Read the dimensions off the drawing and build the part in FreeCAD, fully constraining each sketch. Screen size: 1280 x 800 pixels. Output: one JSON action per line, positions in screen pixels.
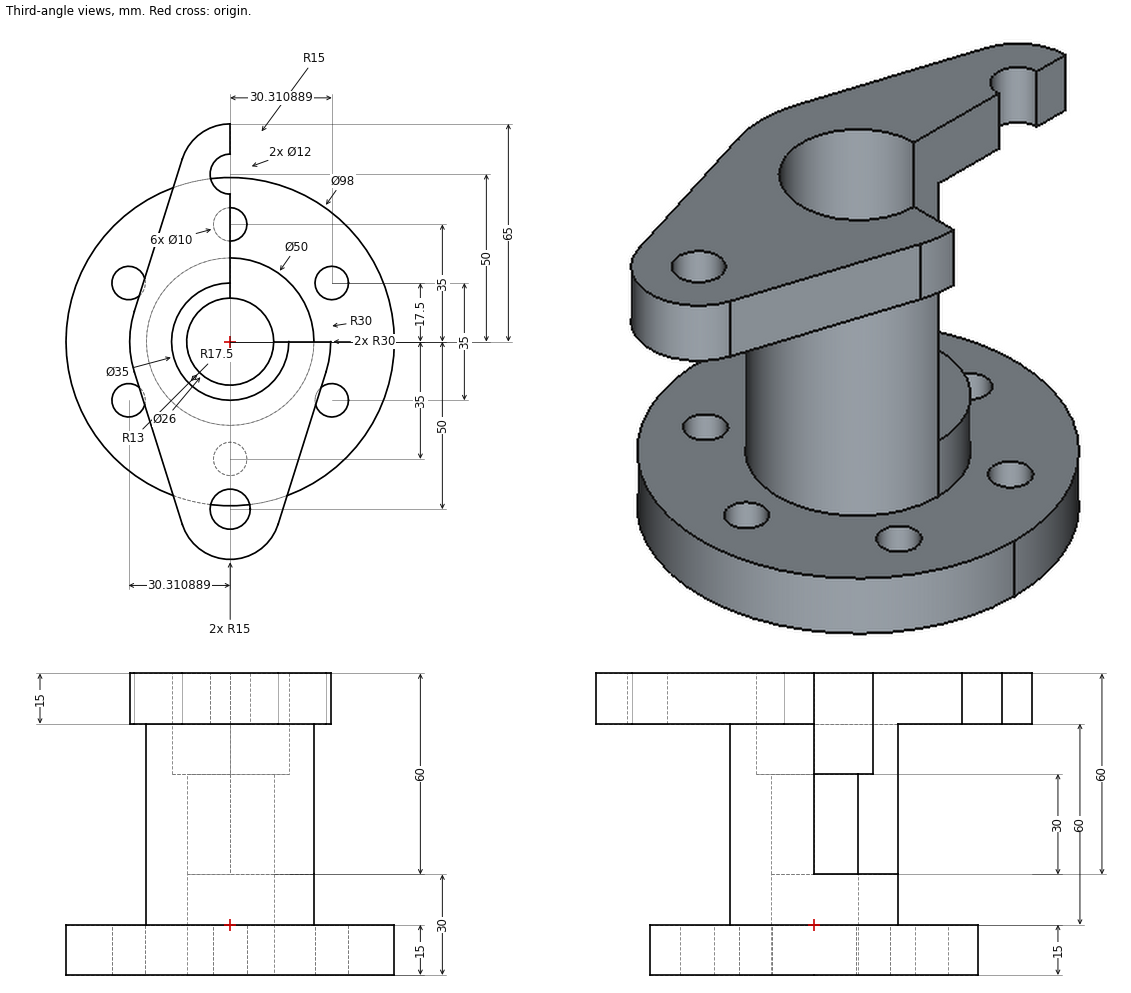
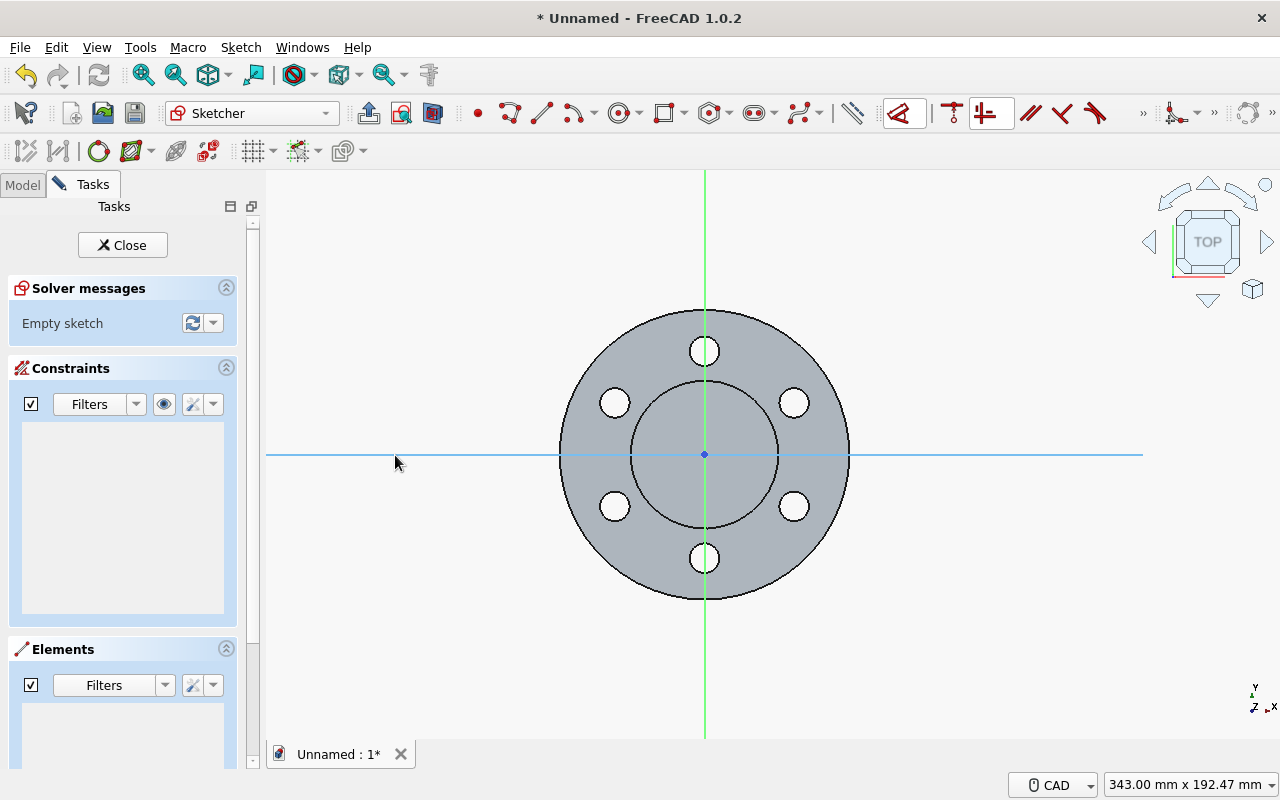
{"action": "left_click", "coordinate": [542, 114]}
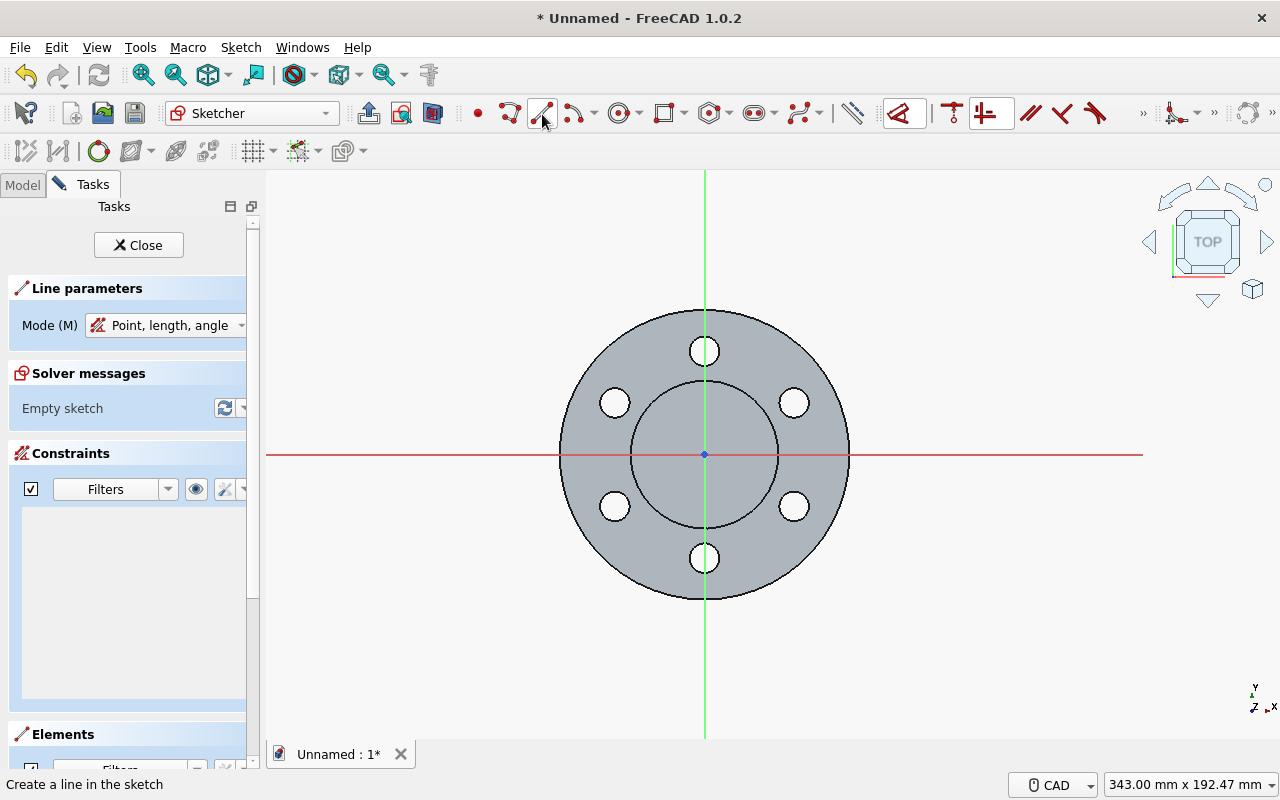
{"action": "left_click", "coordinate": [620, 481]}
{"action": "left_click", "coordinate": [662, 616]}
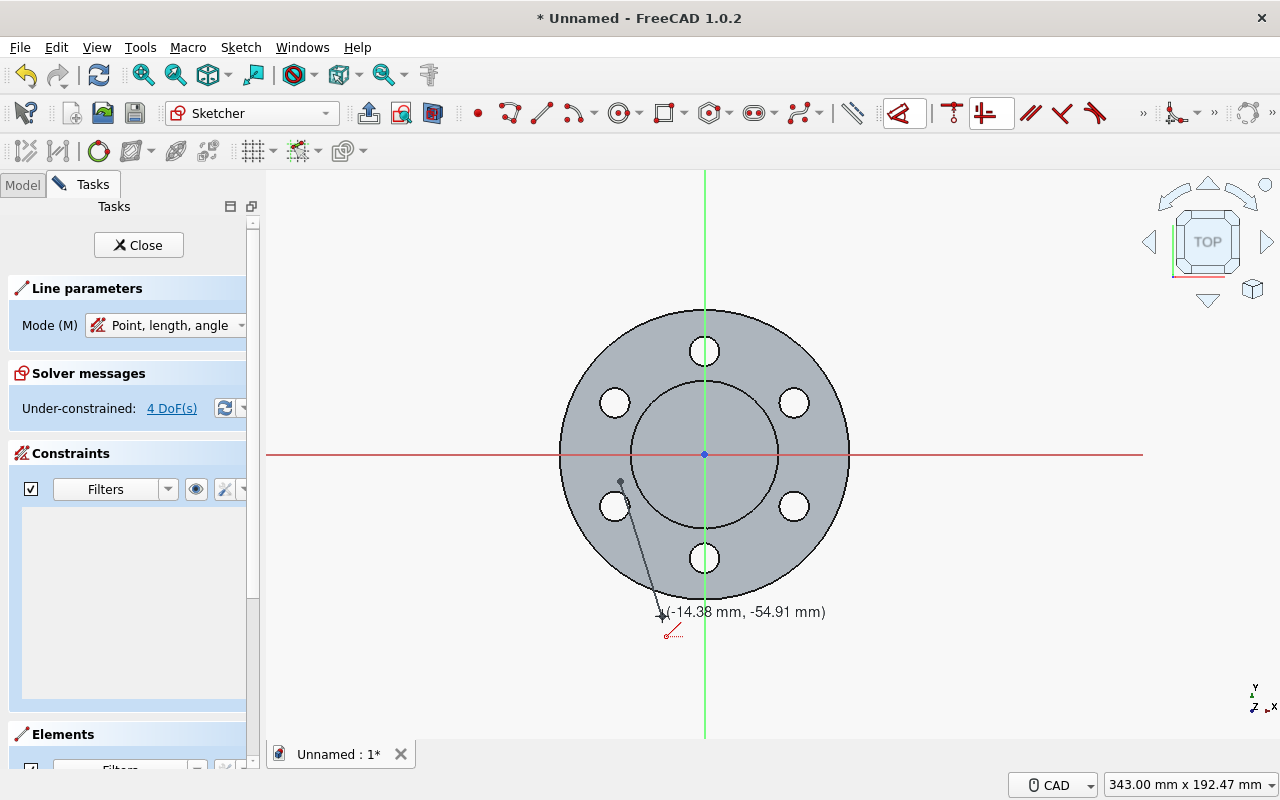
{"action": "left_click", "coordinate": [747, 616]}
{"action": "left_click", "coordinate": [789, 481]}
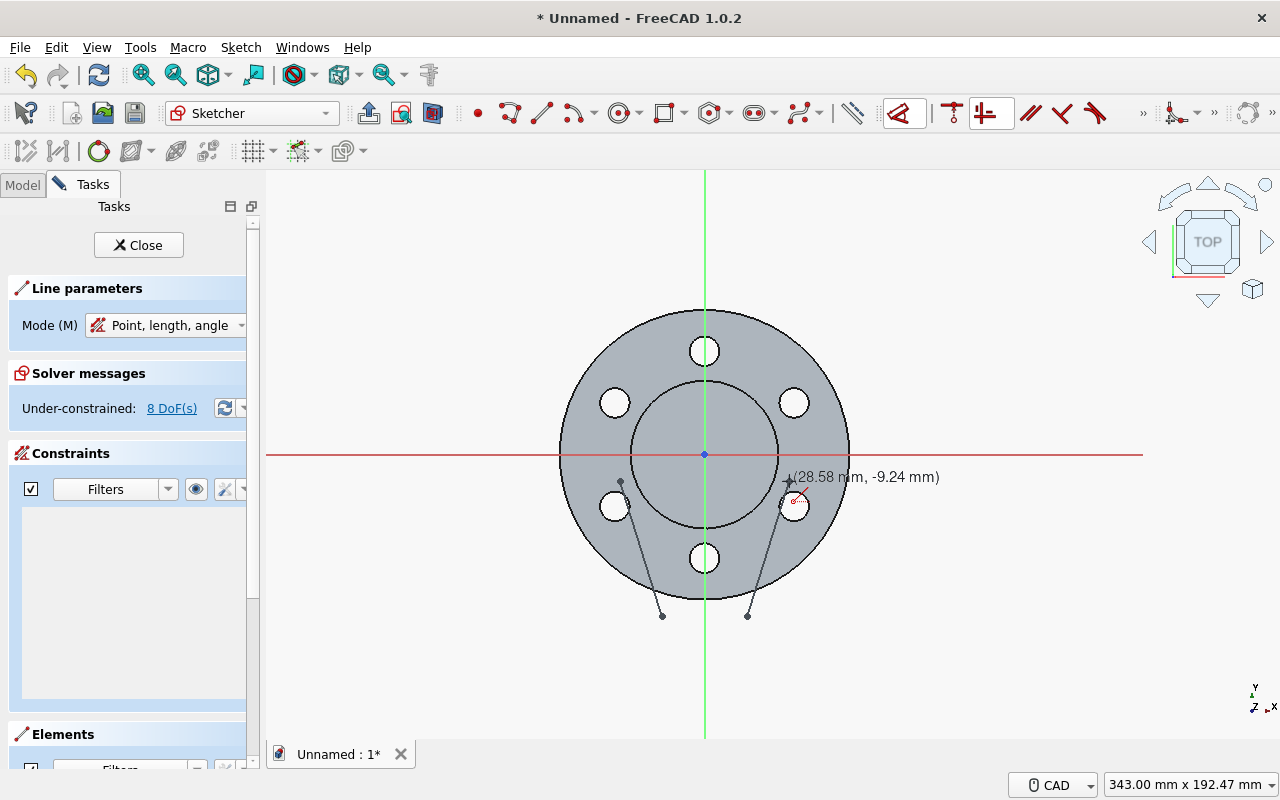
{"action": "left_click", "coordinate": [789, 428]}
{"action": "left_click", "coordinate": [747, 294]}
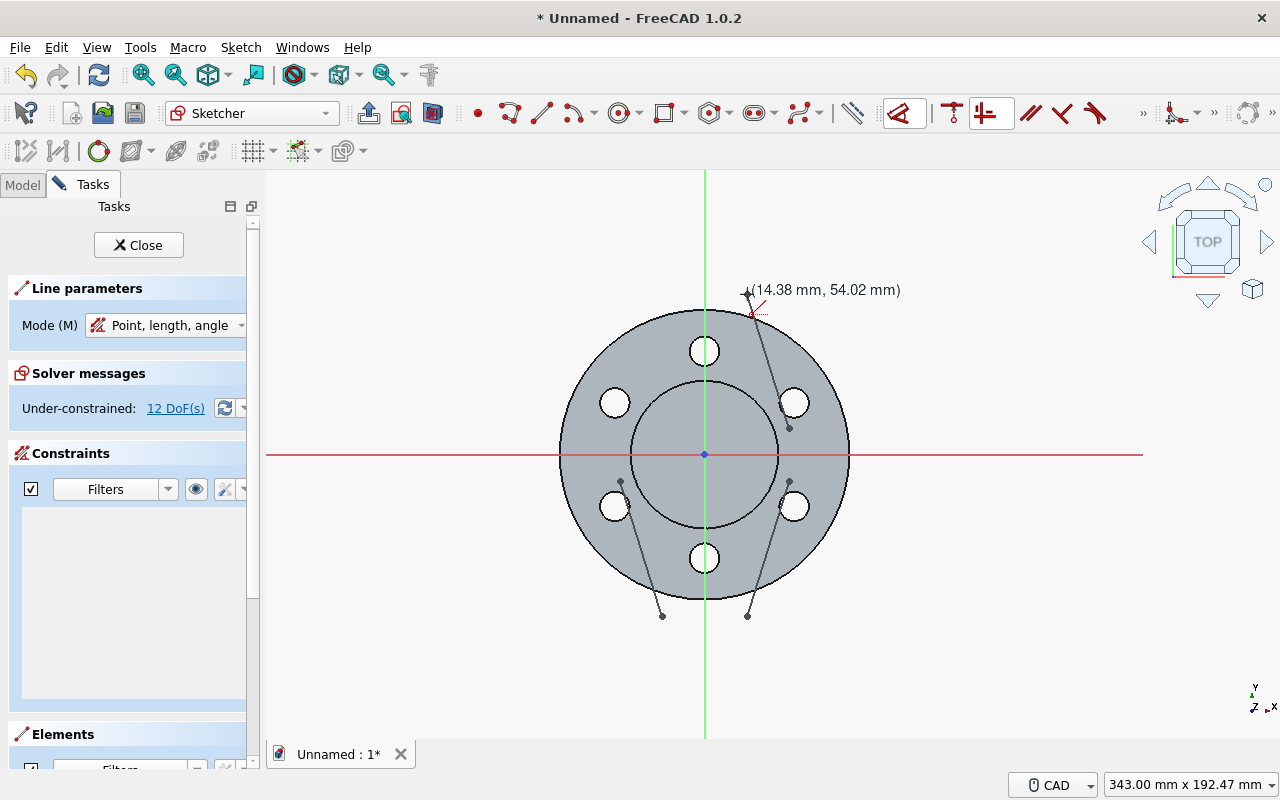
{"action": "left_click", "coordinate": [662, 294]}
{"action": "left_click", "coordinate": [620, 428]}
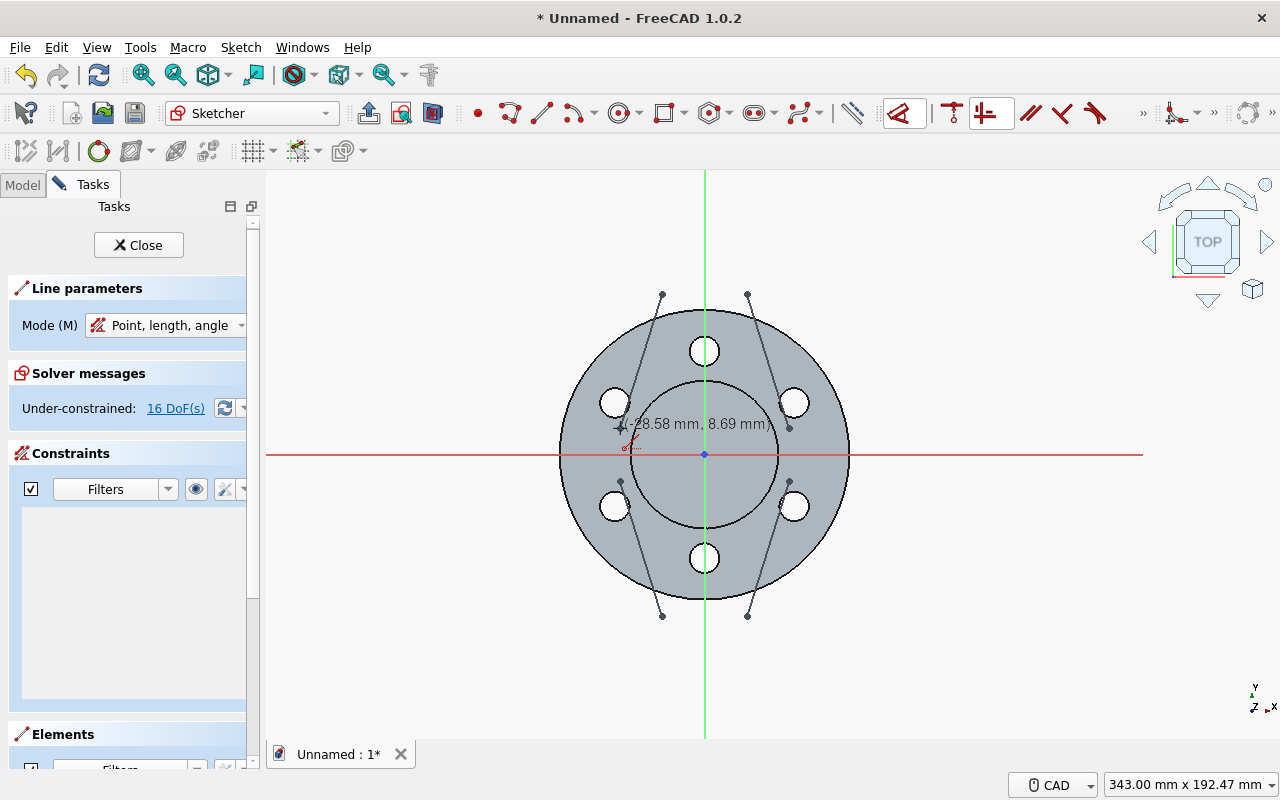
{"action": "left_click", "coordinate": [596, 114]}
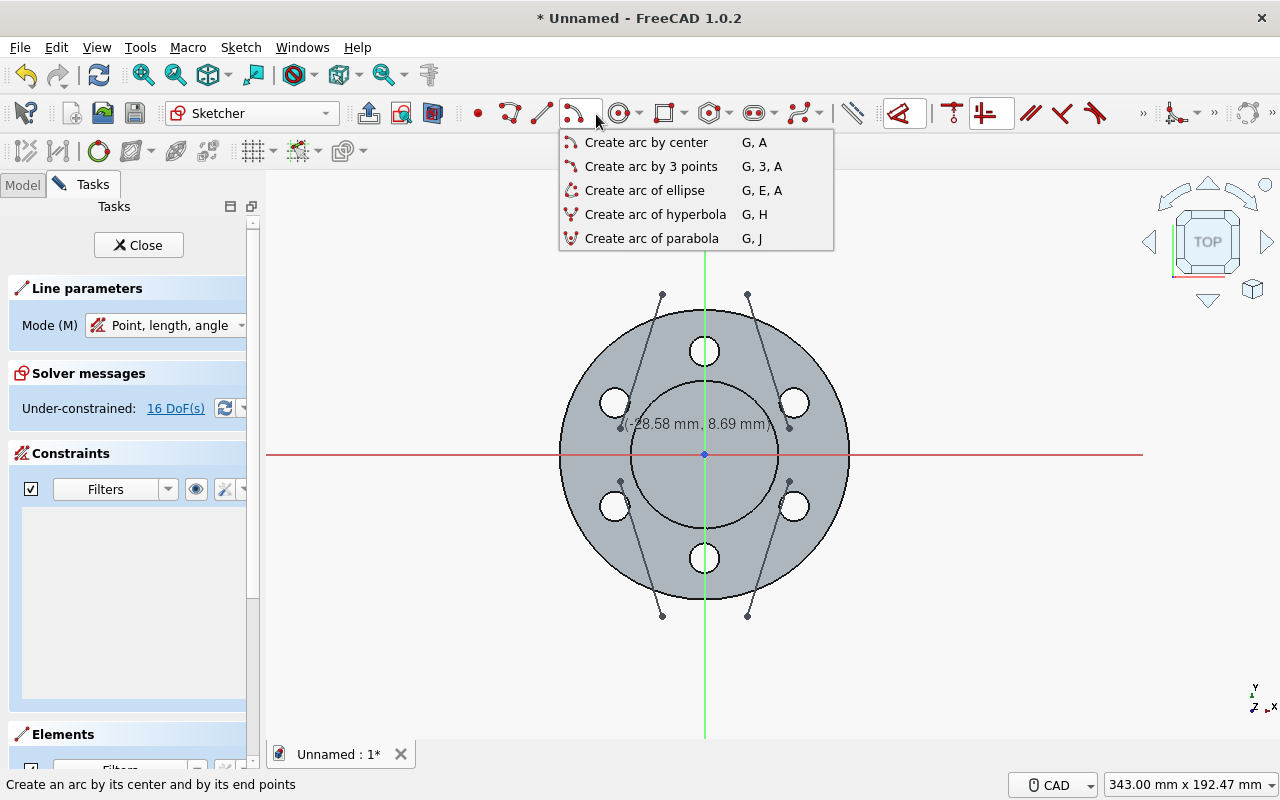
{"action": "left_click", "coordinate": [696, 166]}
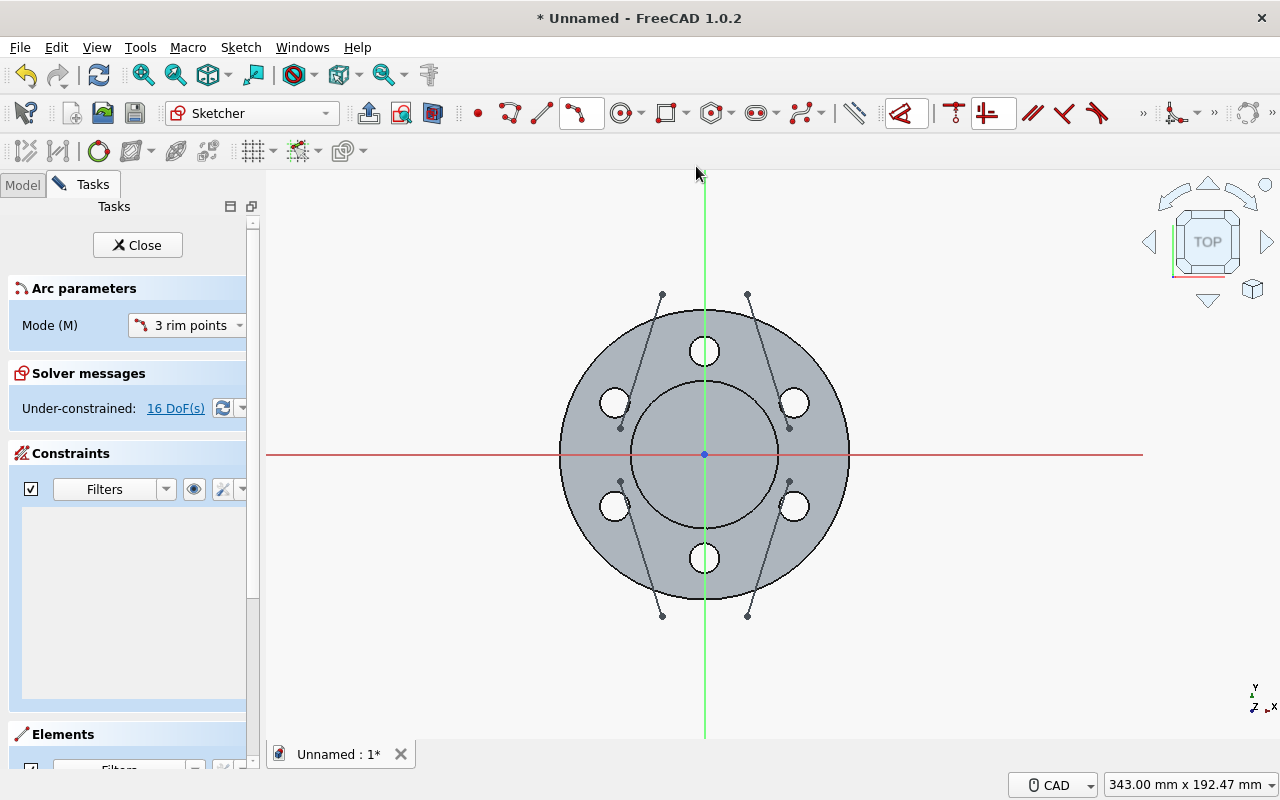
{"action": "left_click", "coordinate": [662, 617]}
{"action": "left_click", "coordinate": [747, 617]}
{"action": "left_click", "coordinate": [683, 641]}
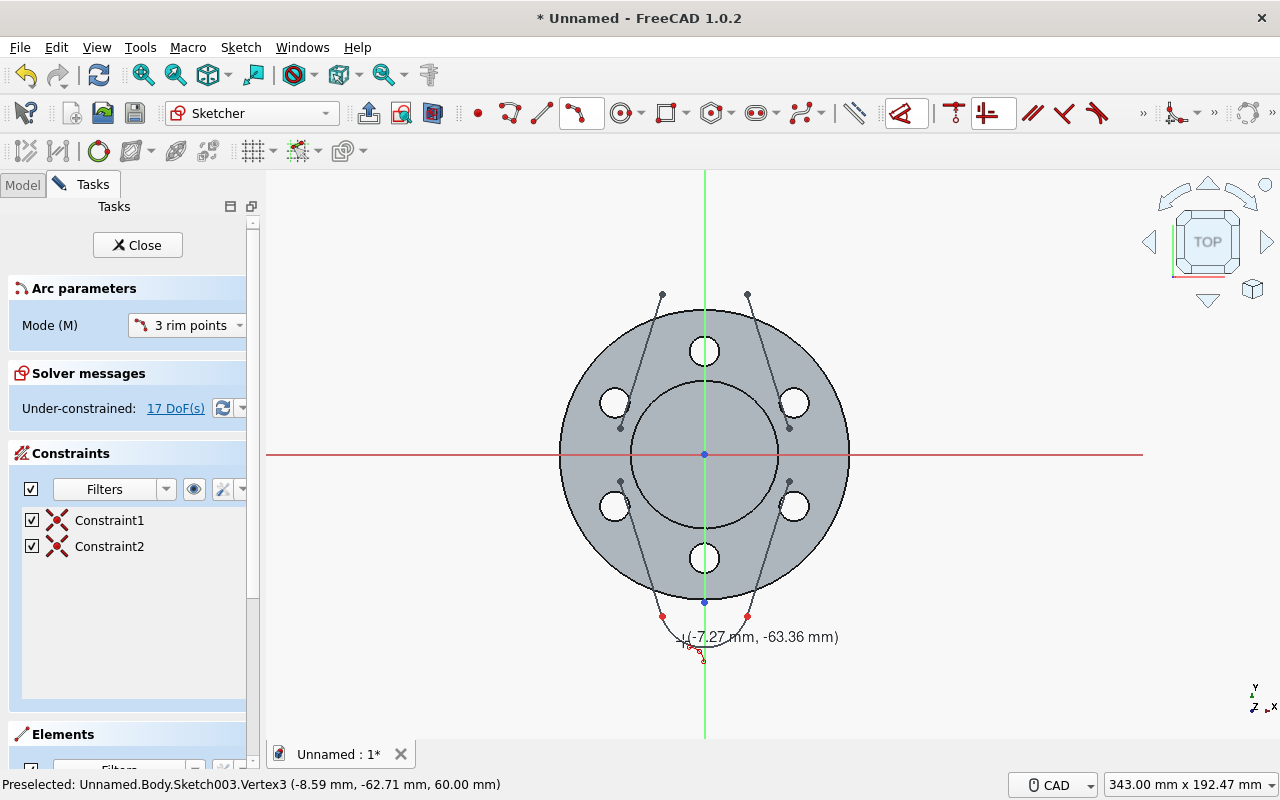
{"action": "left_click", "coordinate": [789, 482]}
{"action": "left_click", "coordinate": [789, 429]}